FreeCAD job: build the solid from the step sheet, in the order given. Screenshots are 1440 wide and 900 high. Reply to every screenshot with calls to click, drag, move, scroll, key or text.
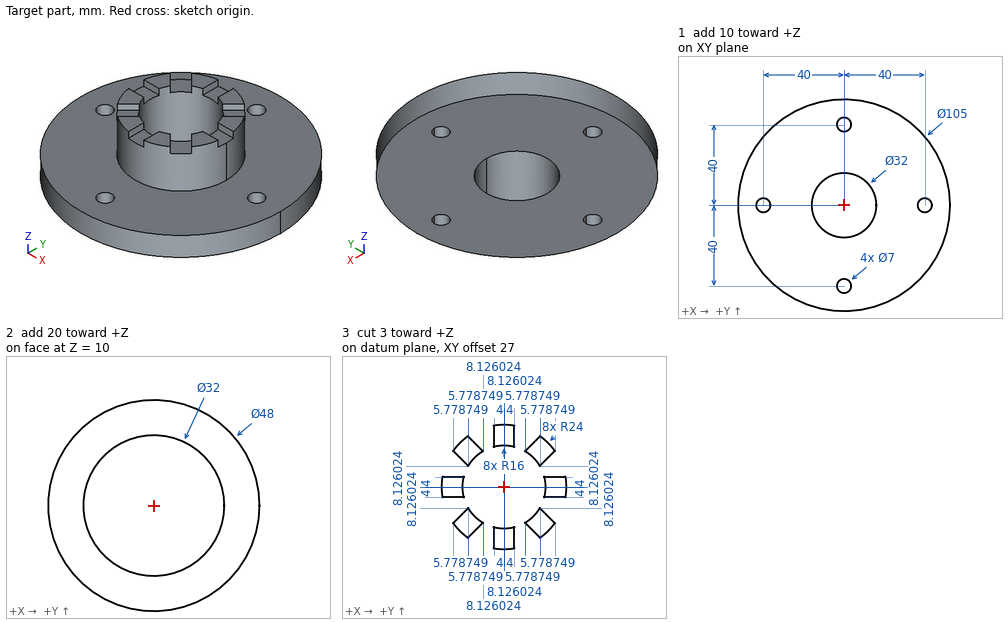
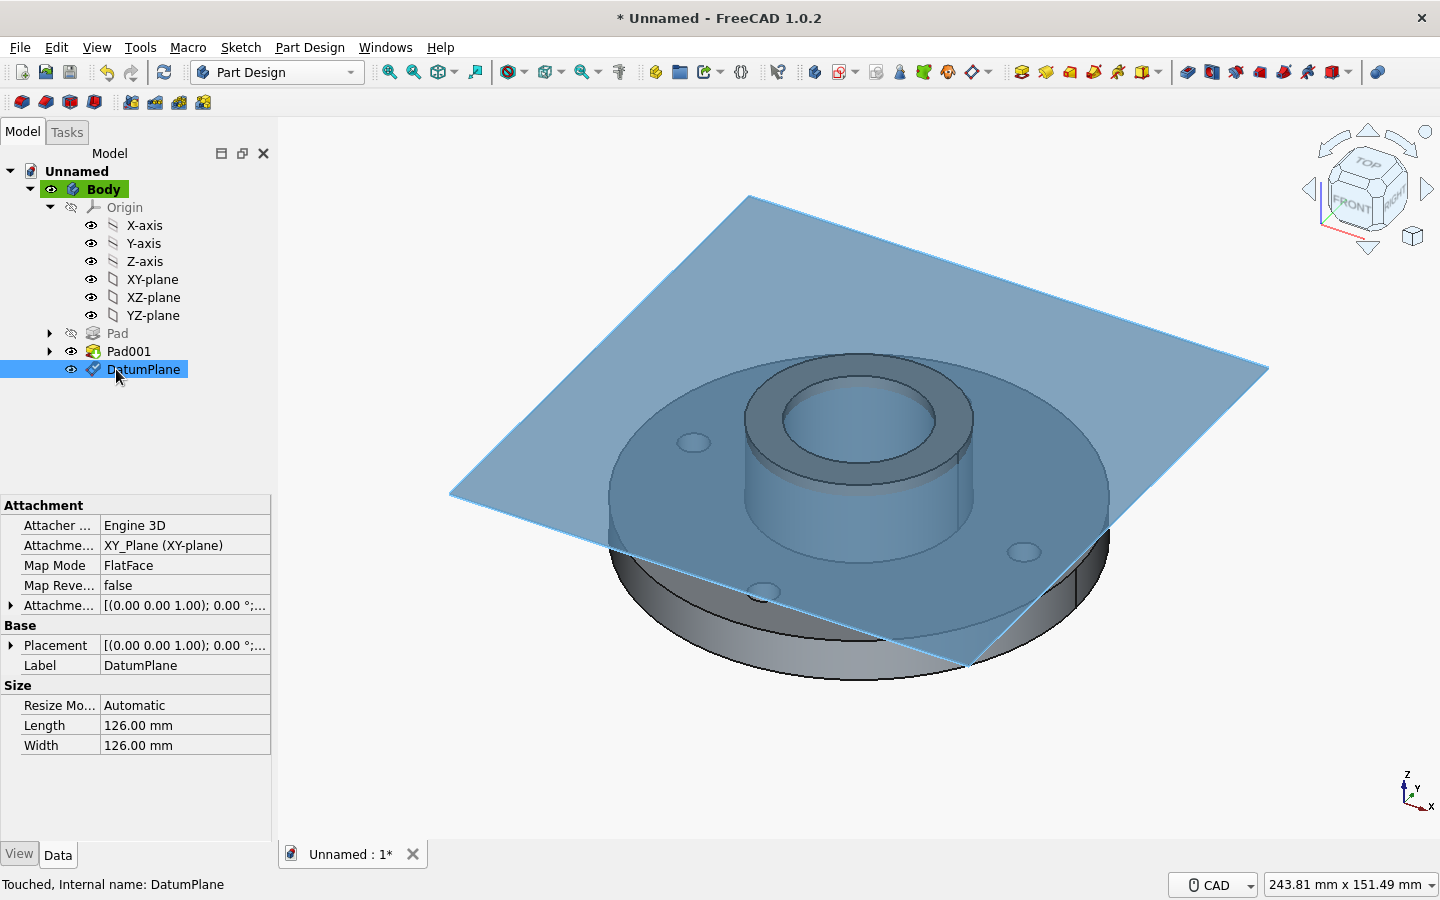
click(840, 72)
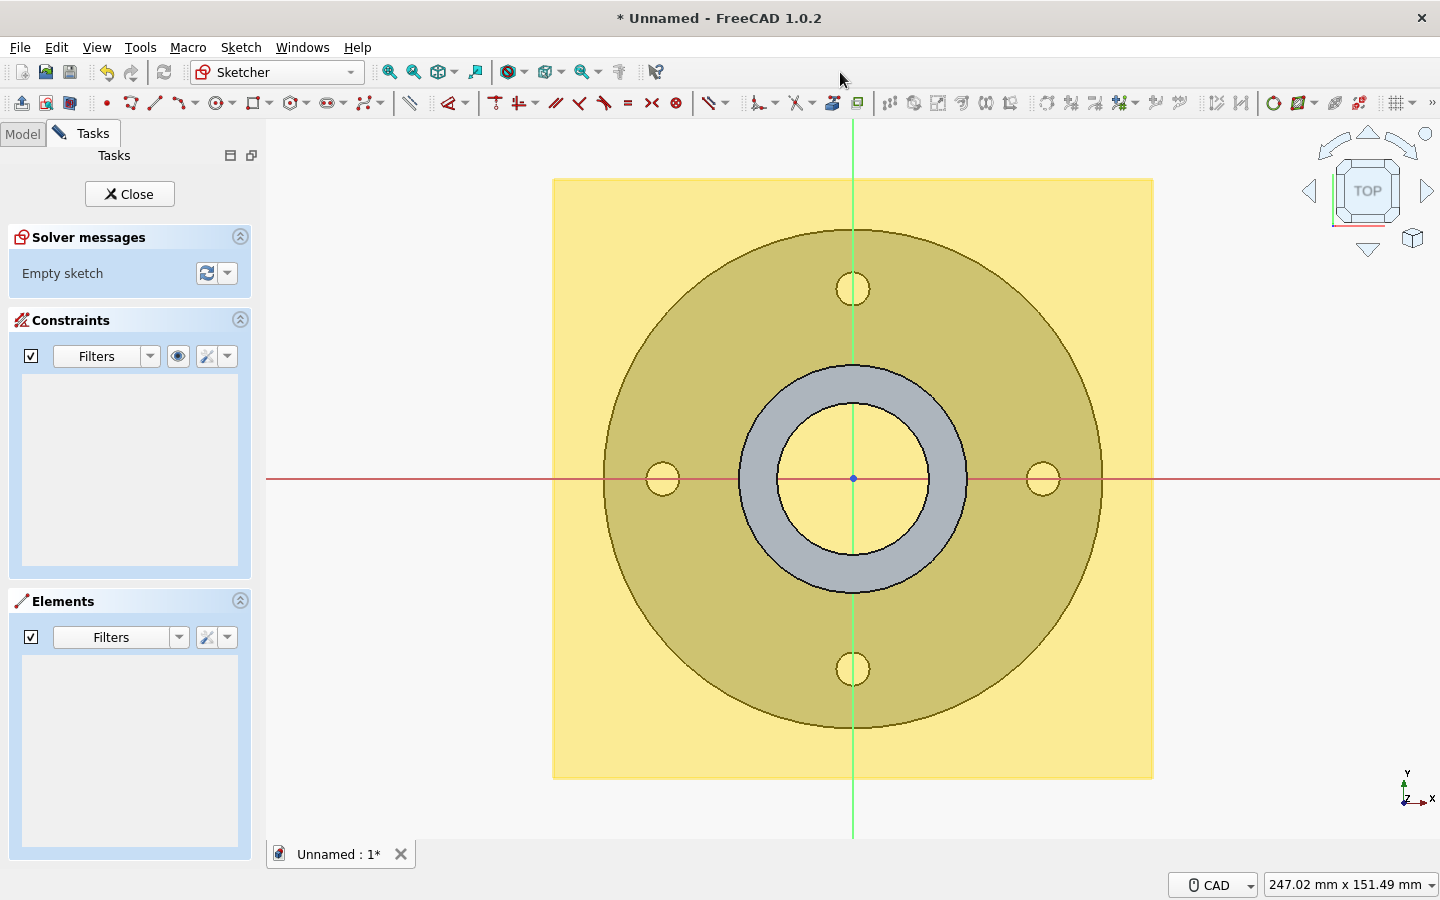
click(70, 104)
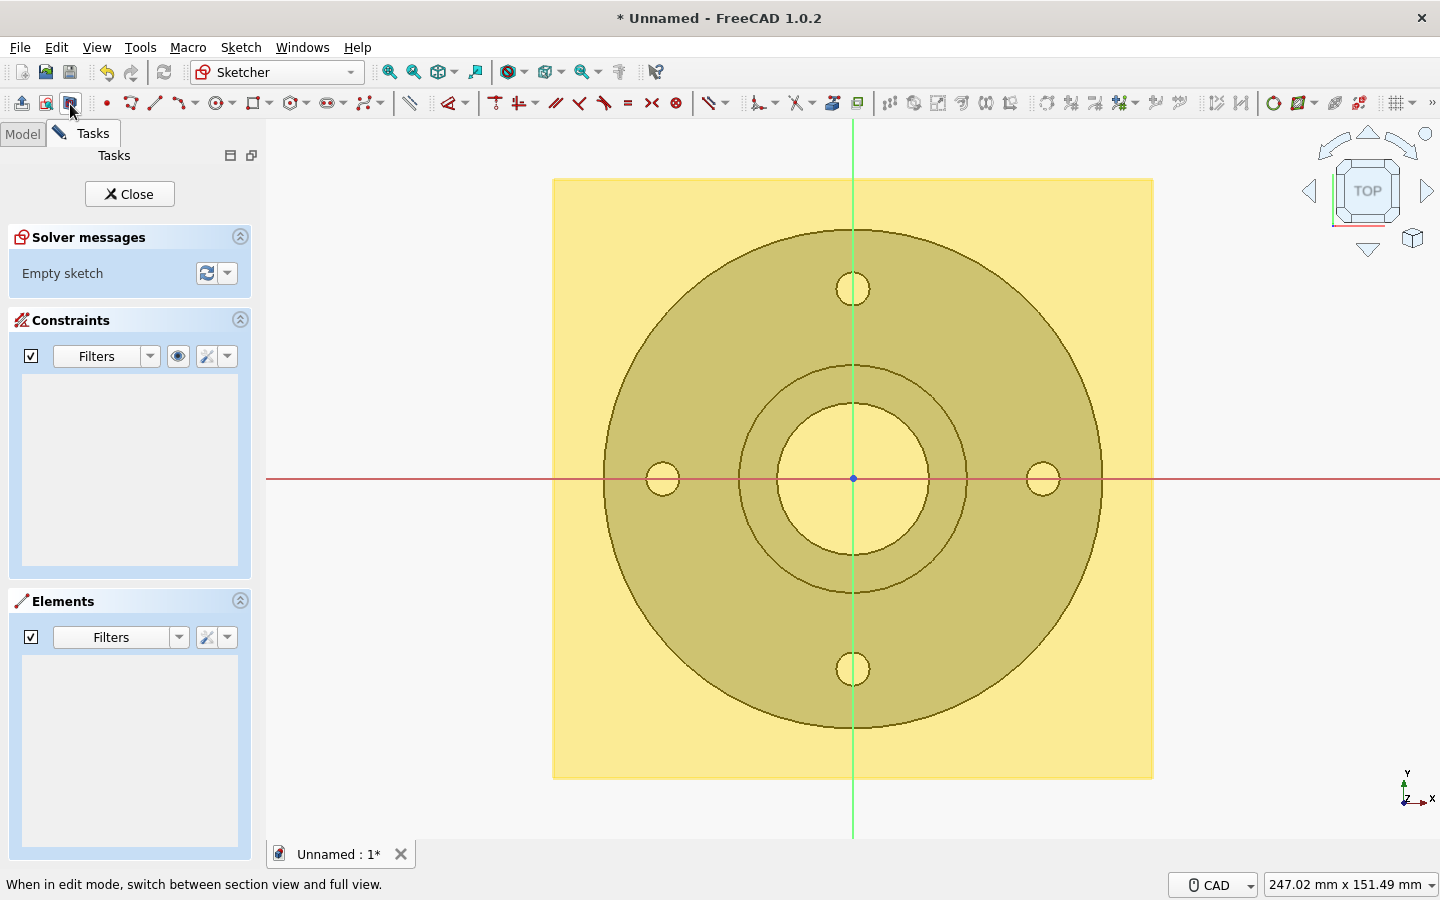
scroll(909, 479, up, 4)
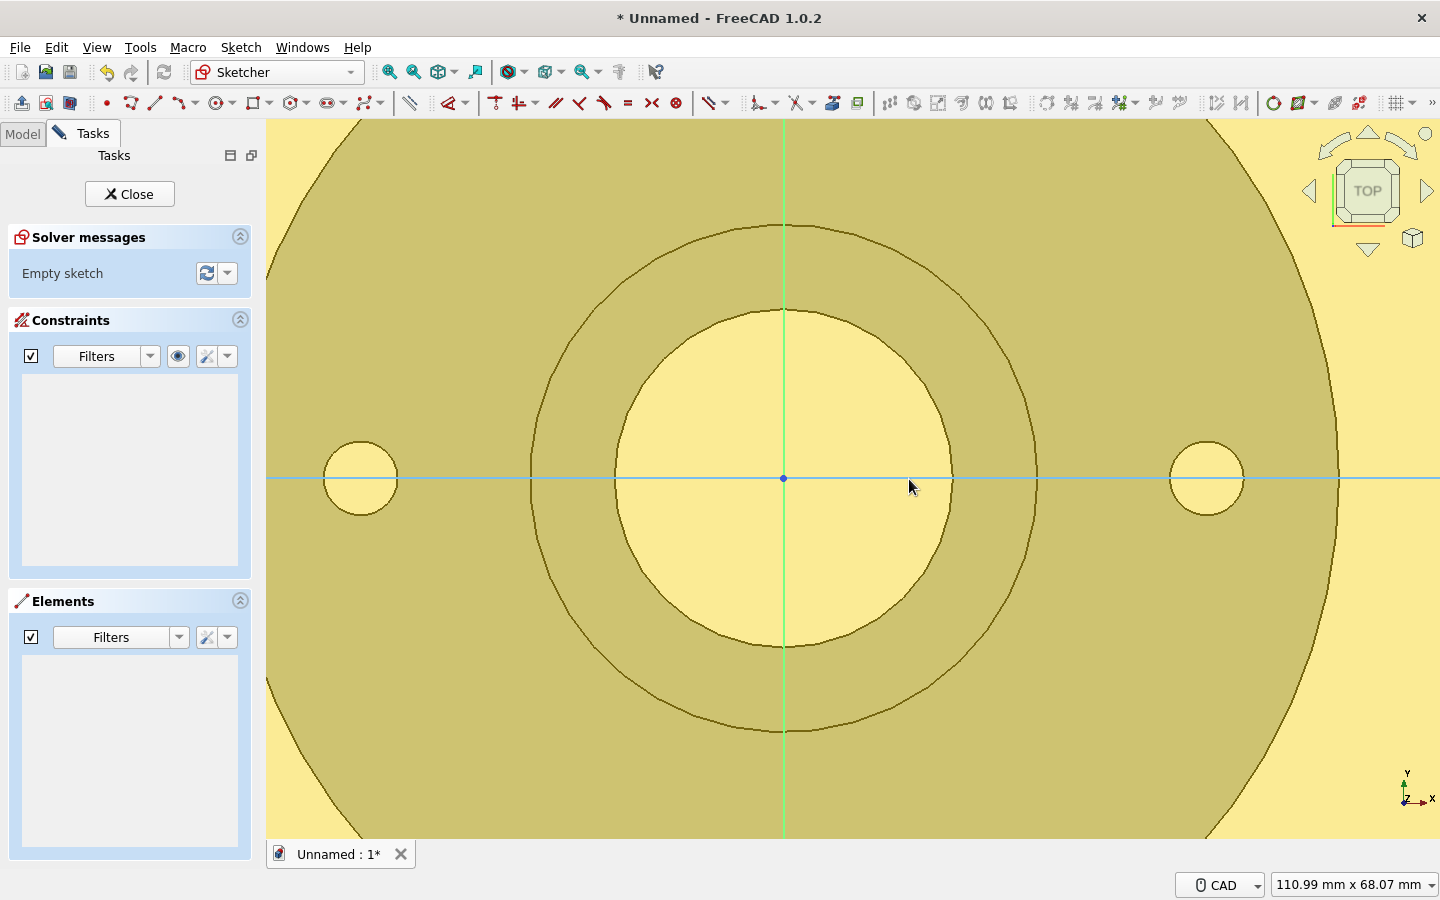
click(156, 104)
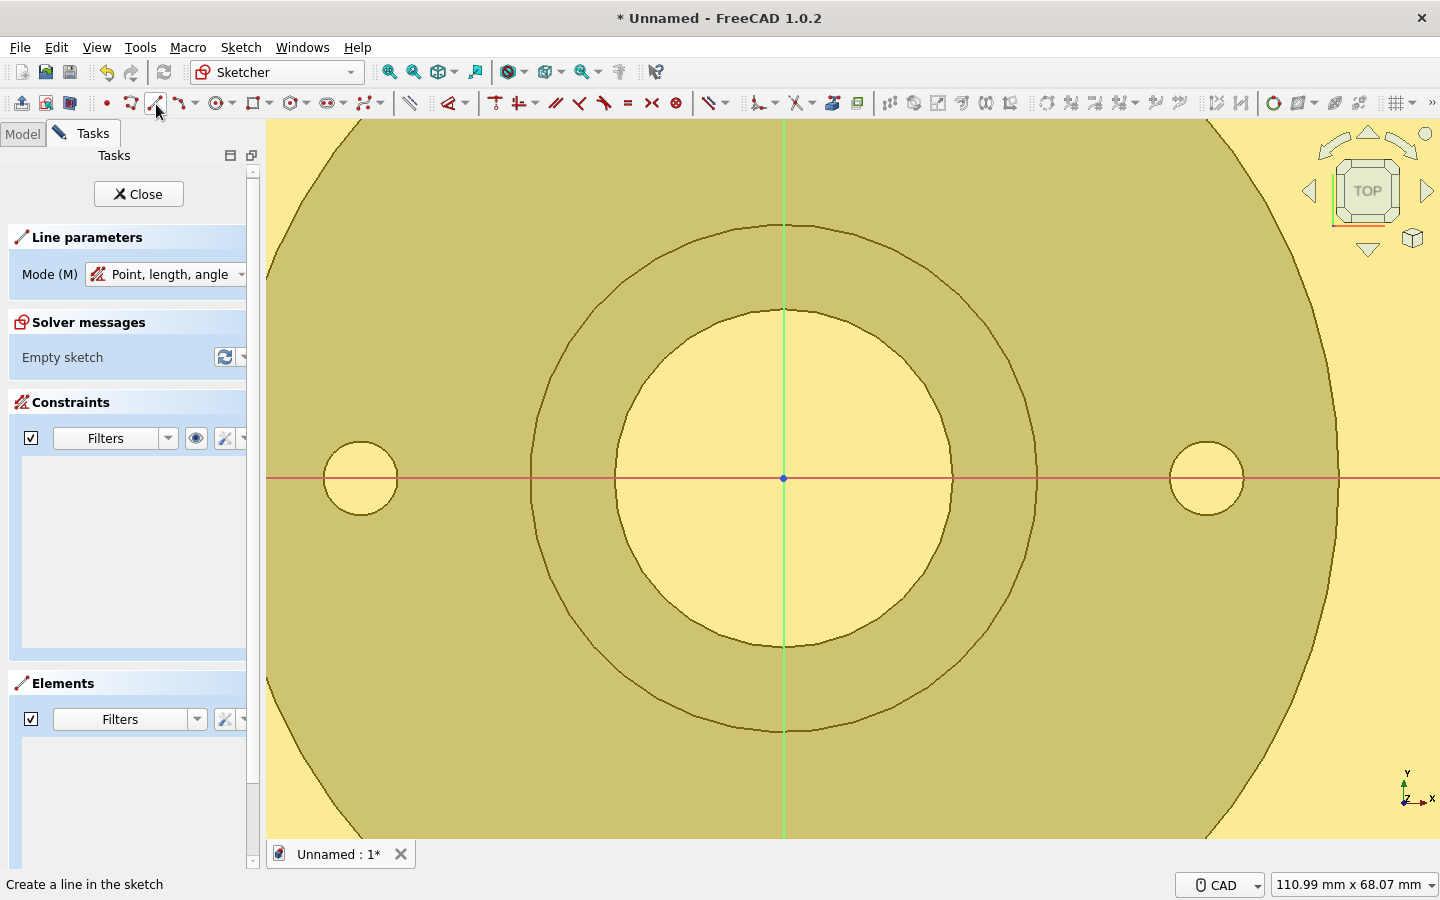
click(741, 228)
click(741, 315)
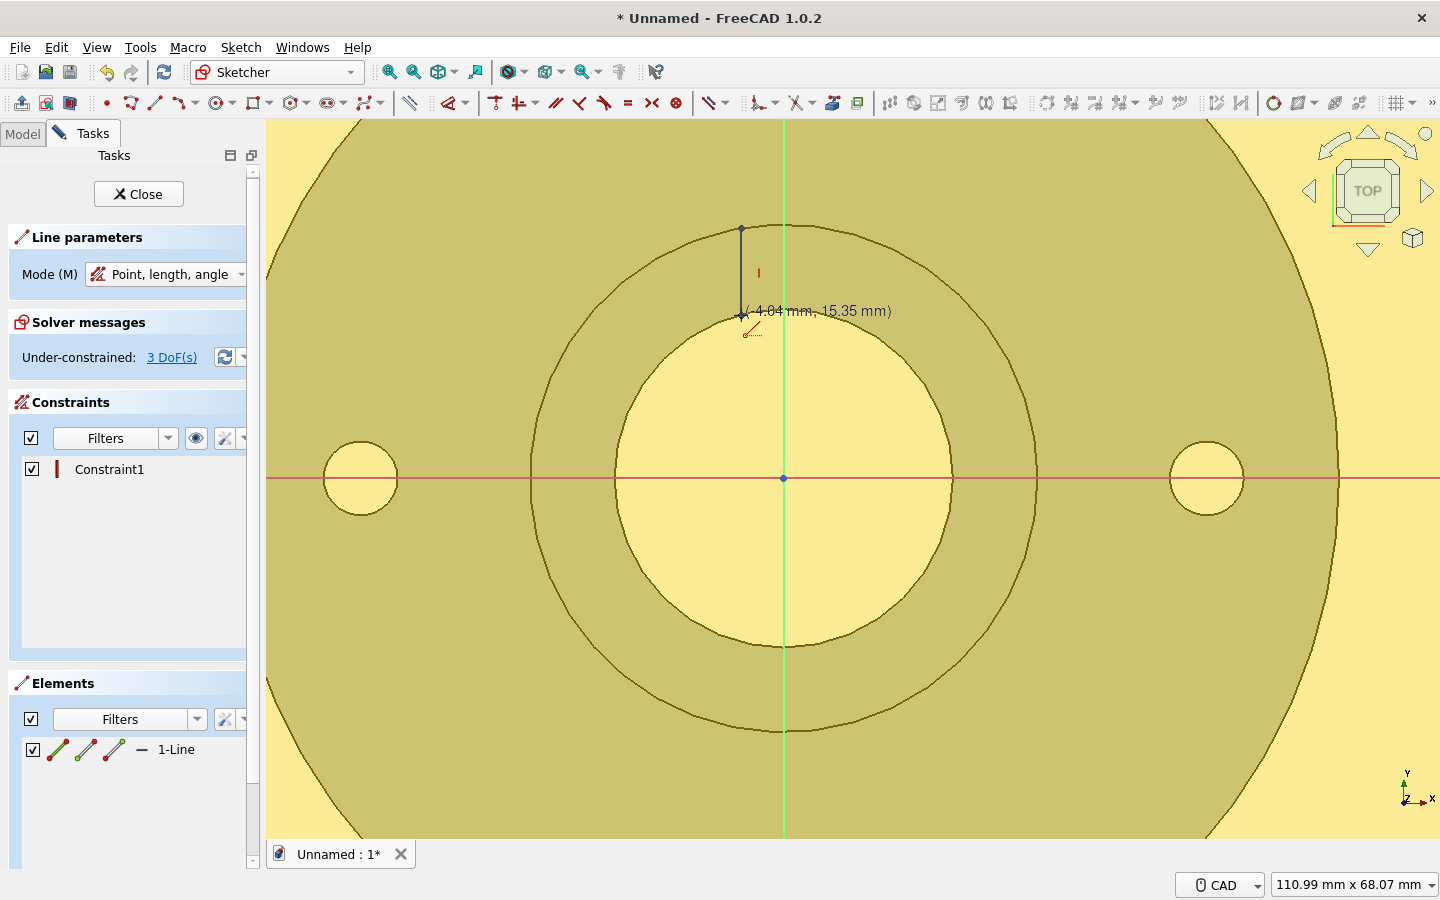
click(826, 315)
click(826, 228)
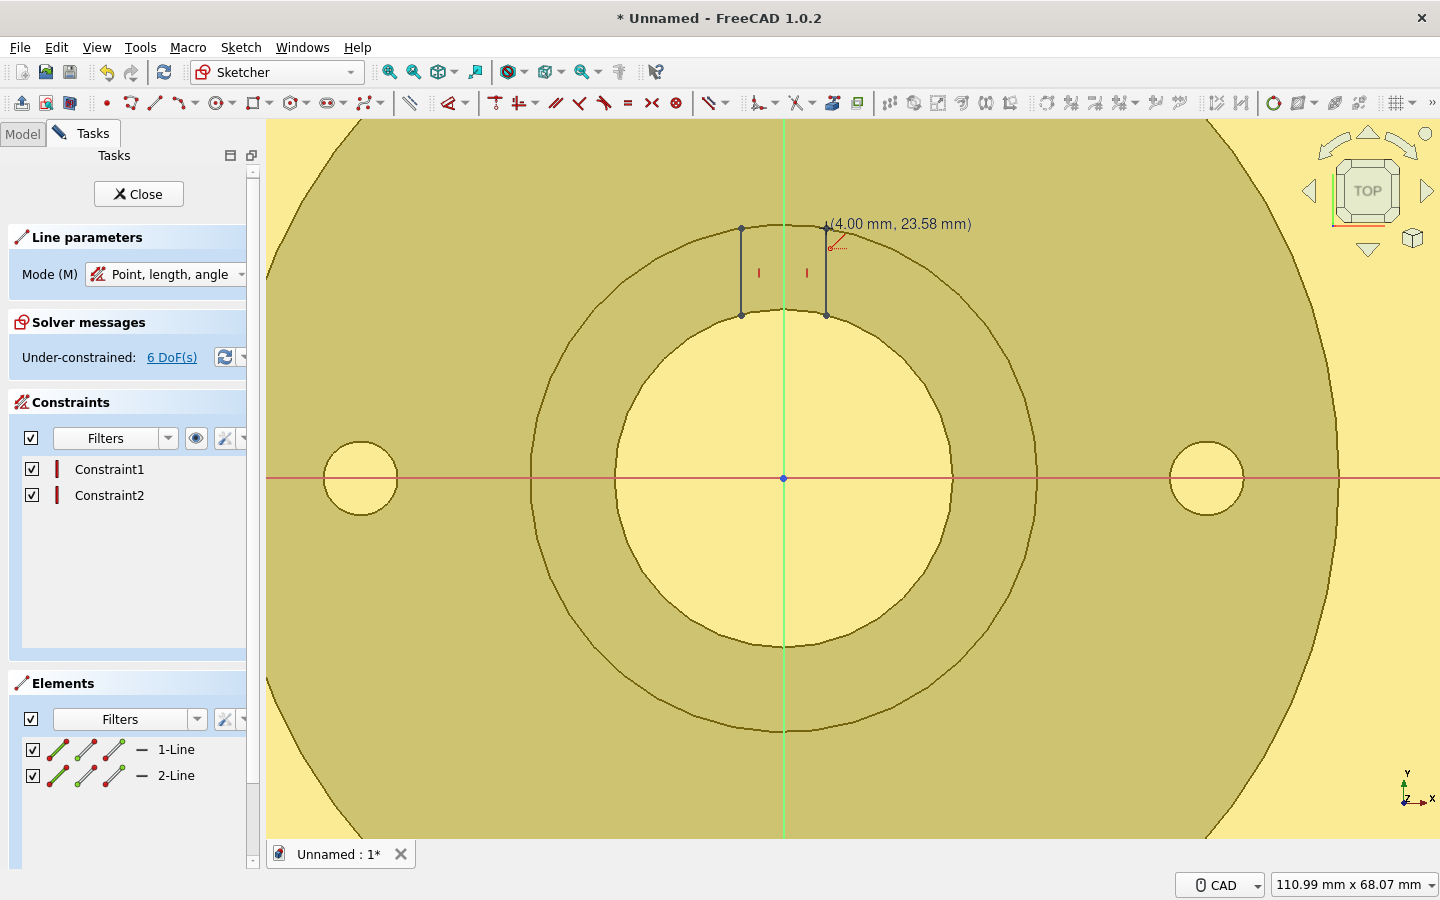
click(180, 104)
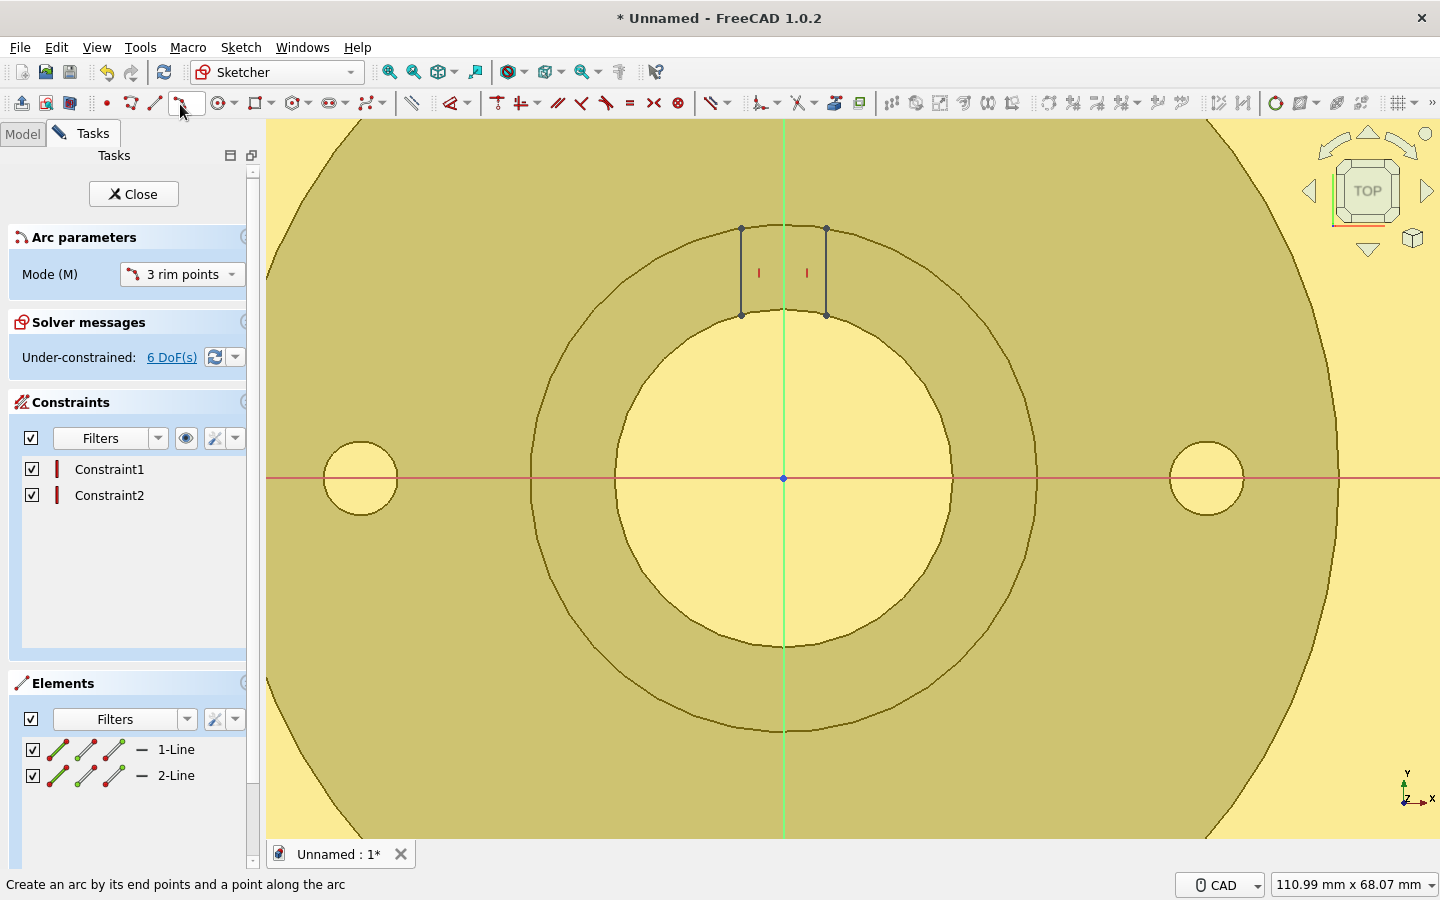
click(741, 316)
click(826, 316)